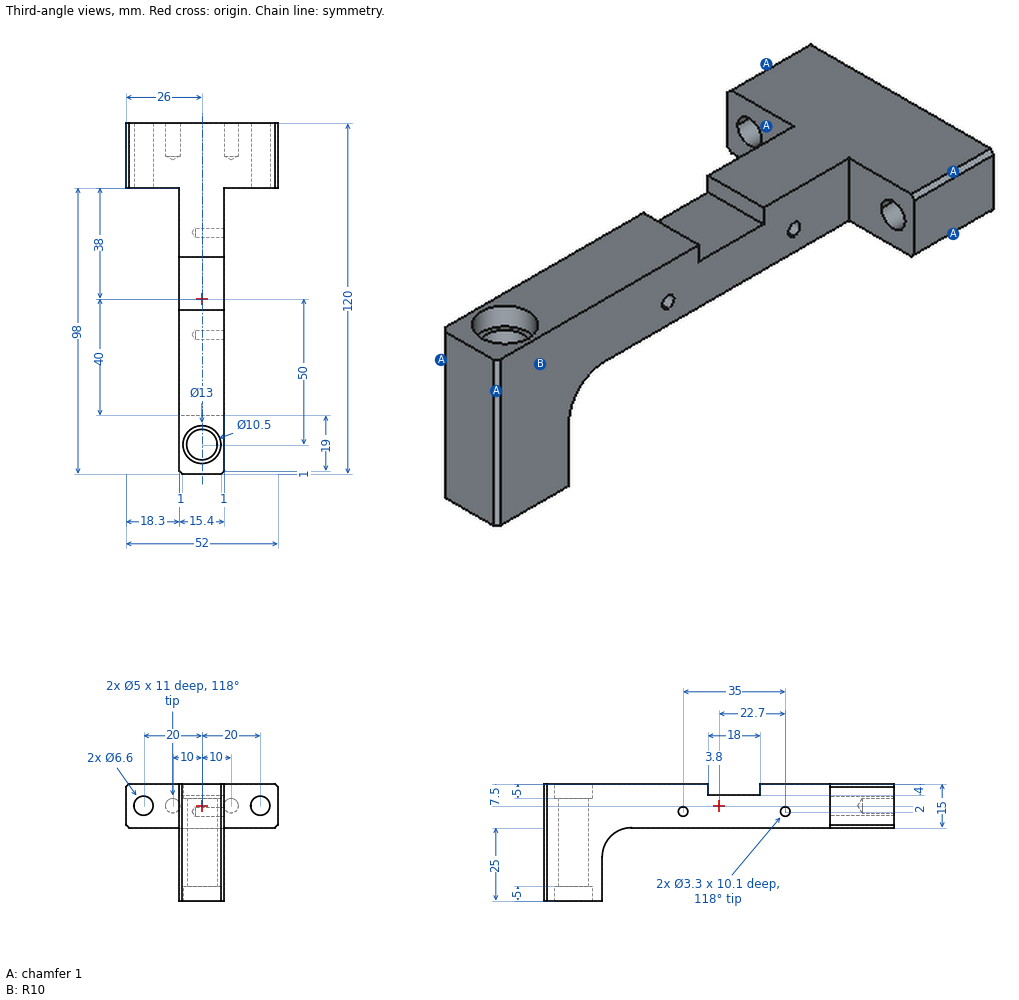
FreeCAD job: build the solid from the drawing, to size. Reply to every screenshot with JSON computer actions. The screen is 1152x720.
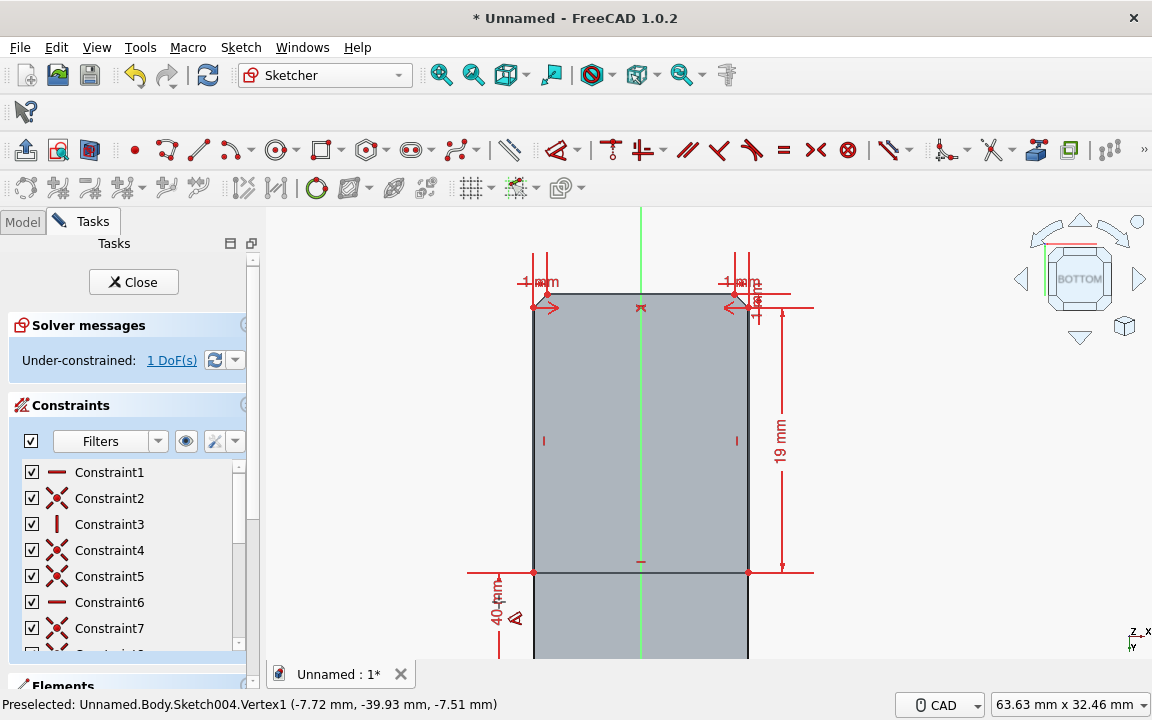
{"action": "left_click", "coordinate": [598, 573]}
{"action": "left_click", "coordinate": [592, 607]}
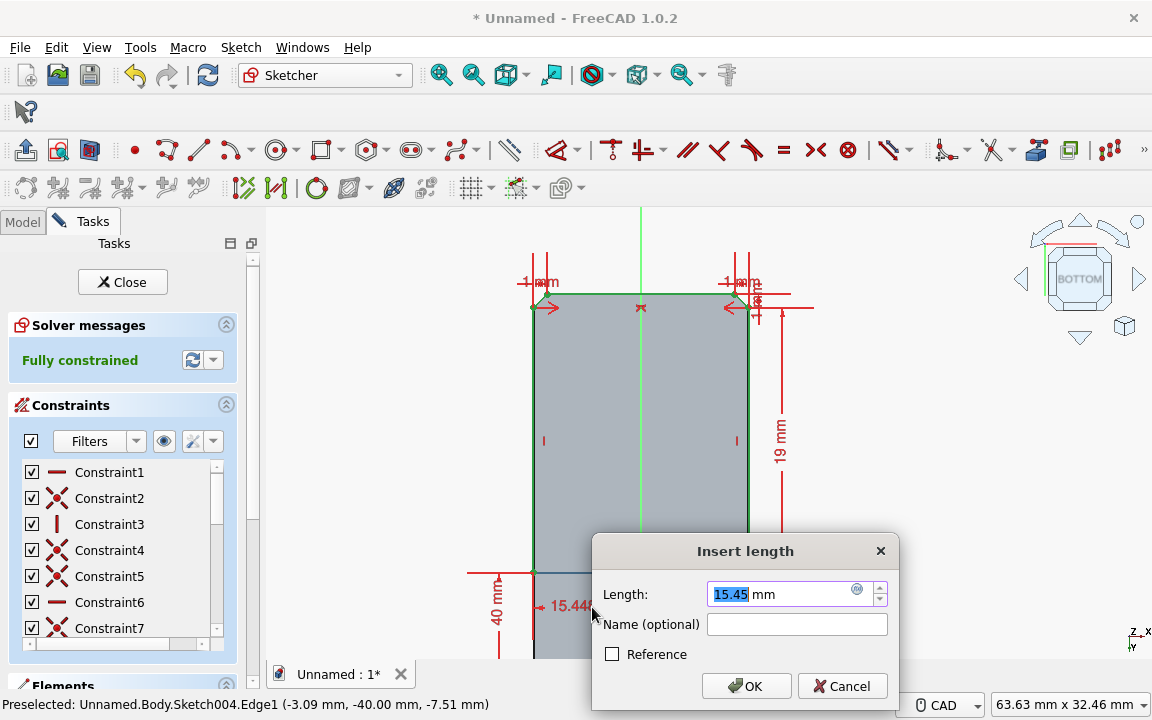
{"action": "type", "text": "15.4"}
{"action": "key", "text": "Return"}
{"action": "key", "text": "Escape"}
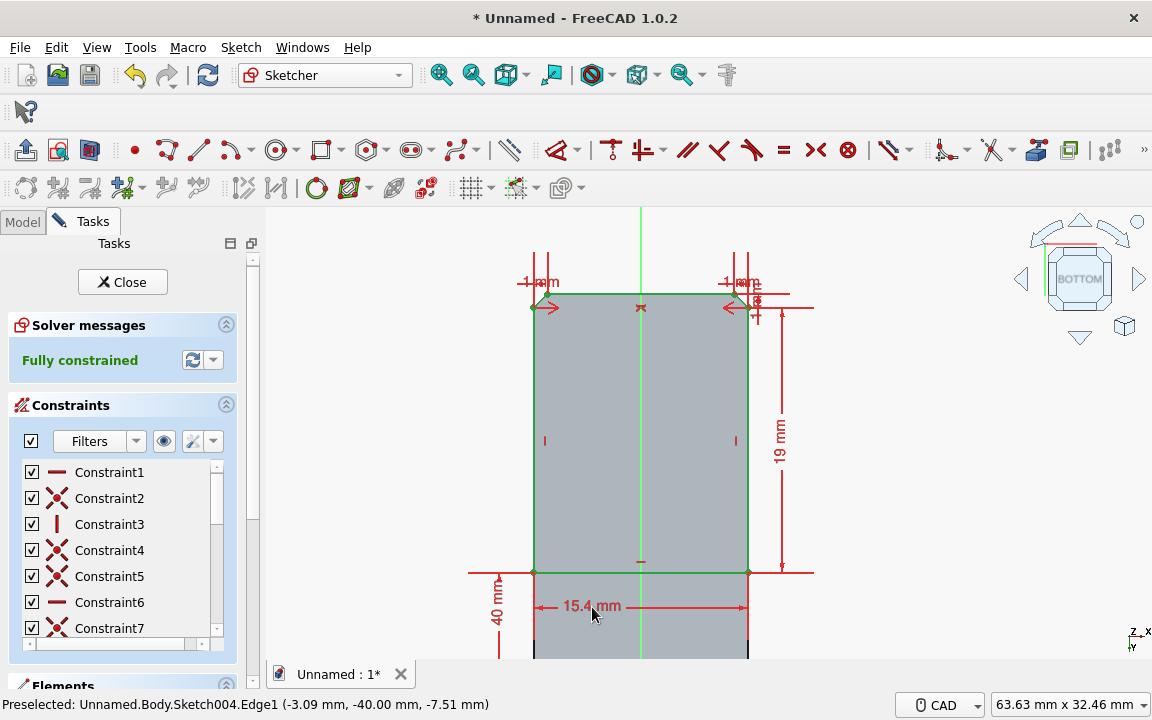
{"action": "left_click", "coordinate": [123, 282]}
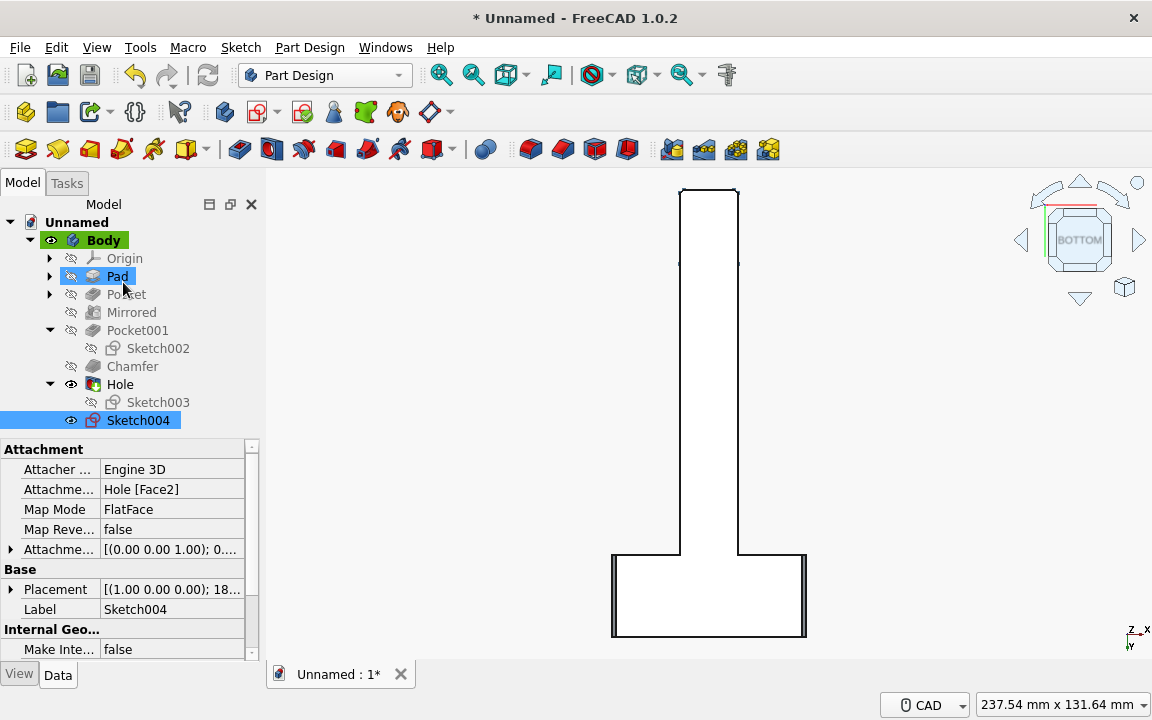
{"action": "left_click", "coordinate": [26, 150]}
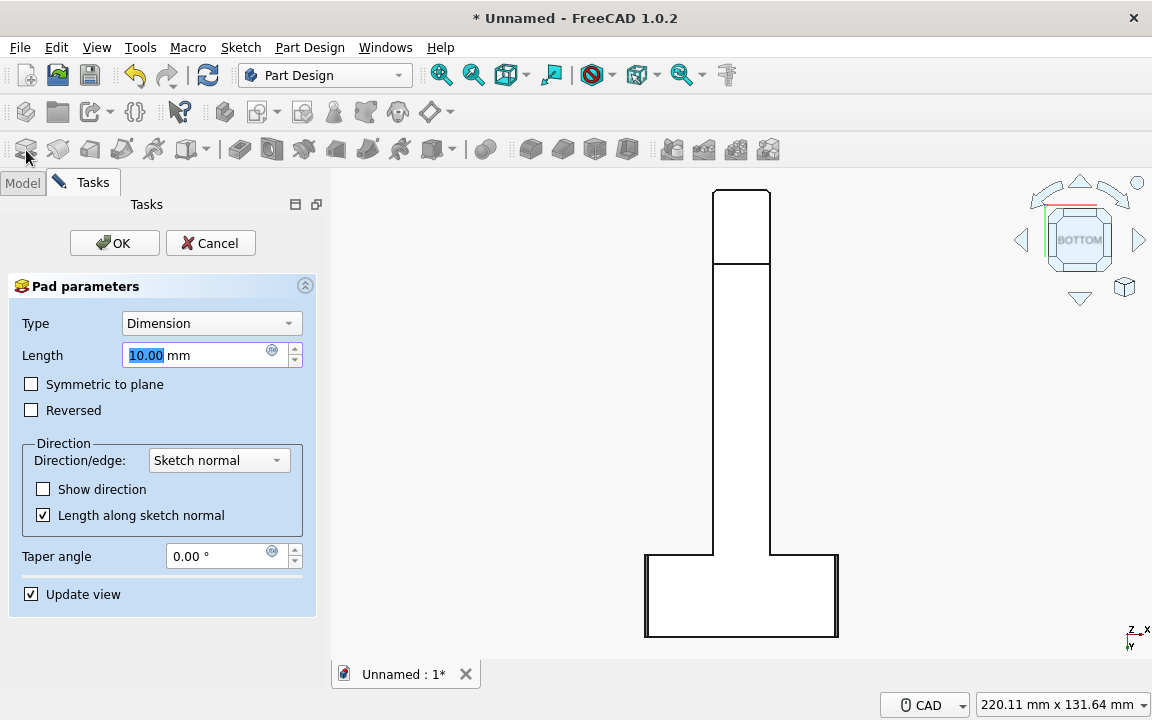
{"action": "type", "text": "25"}
{"action": "key", "text": "Tab"}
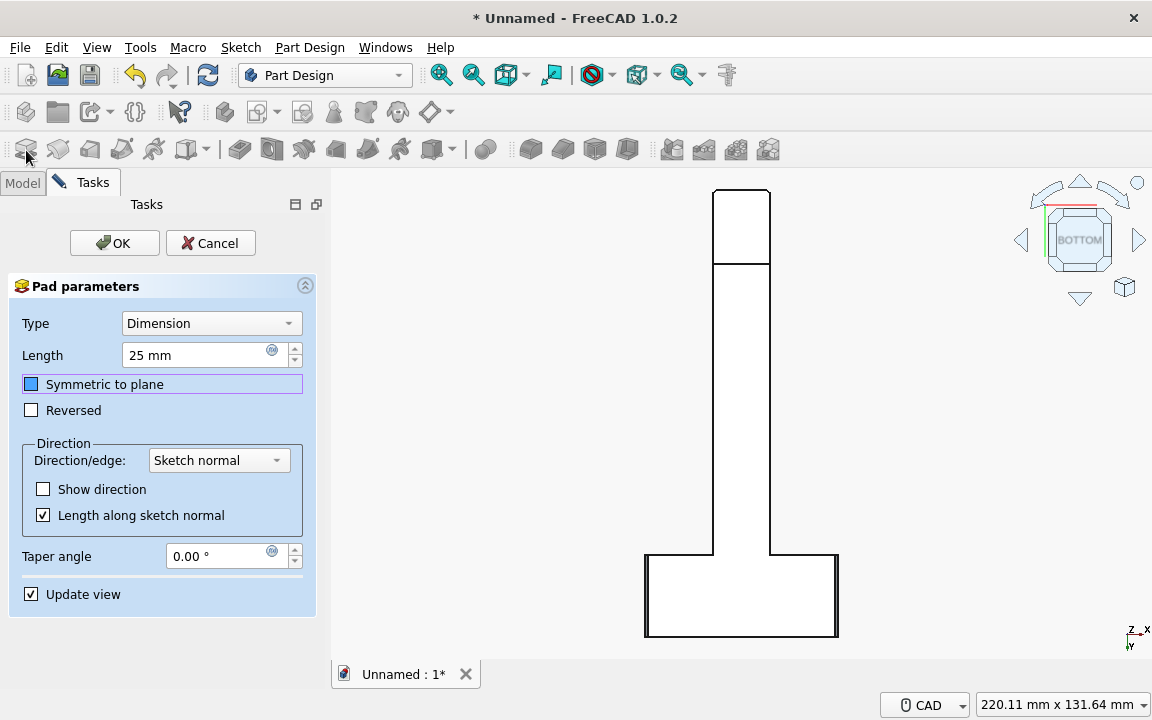
{"action": "left_click", "coordinate": [115, 243]}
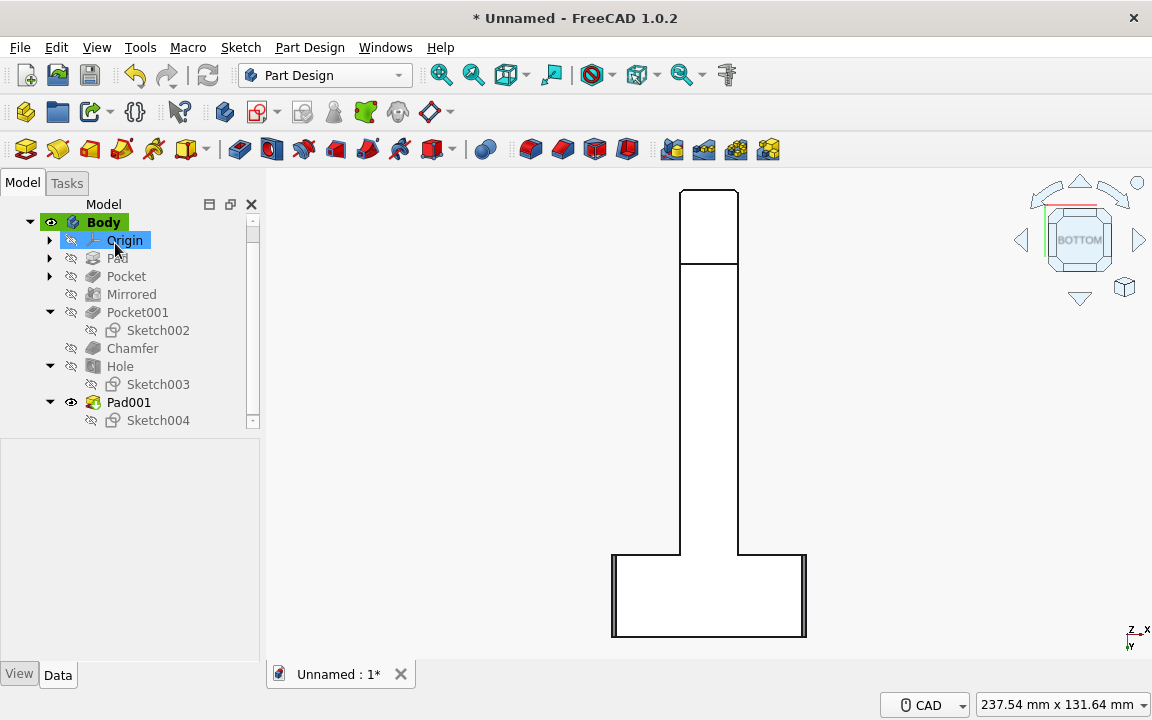
{"action": "key", "text": "0"}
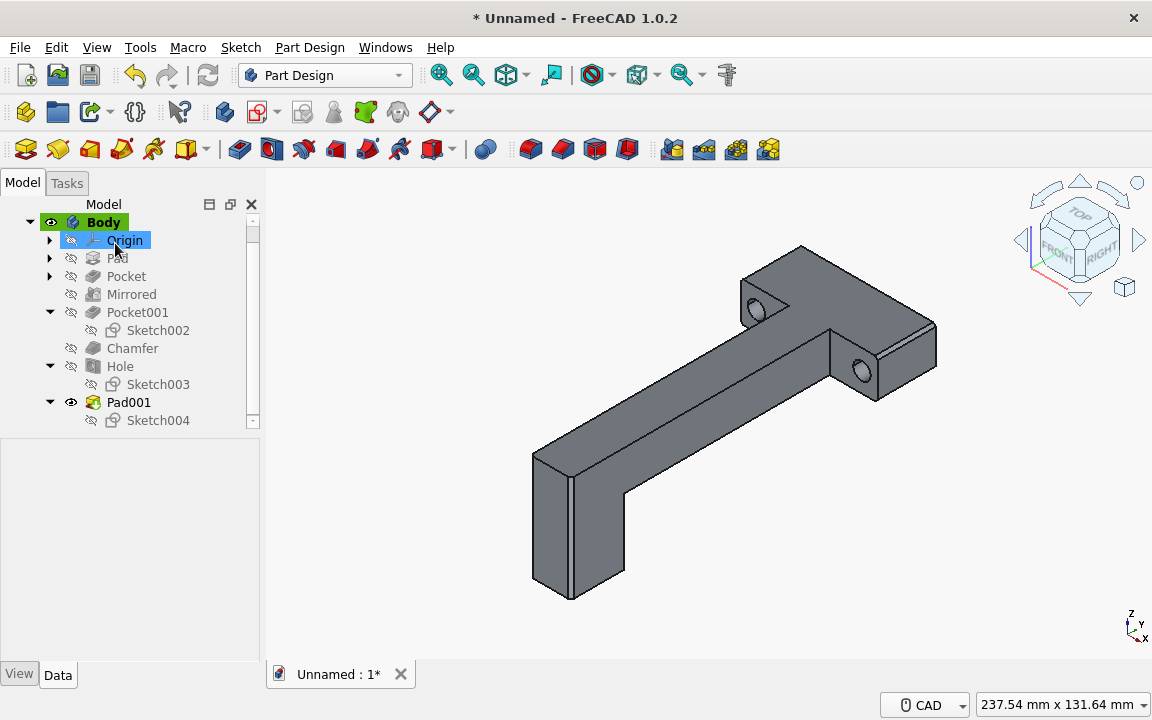
{"action": "key", "text": "2"}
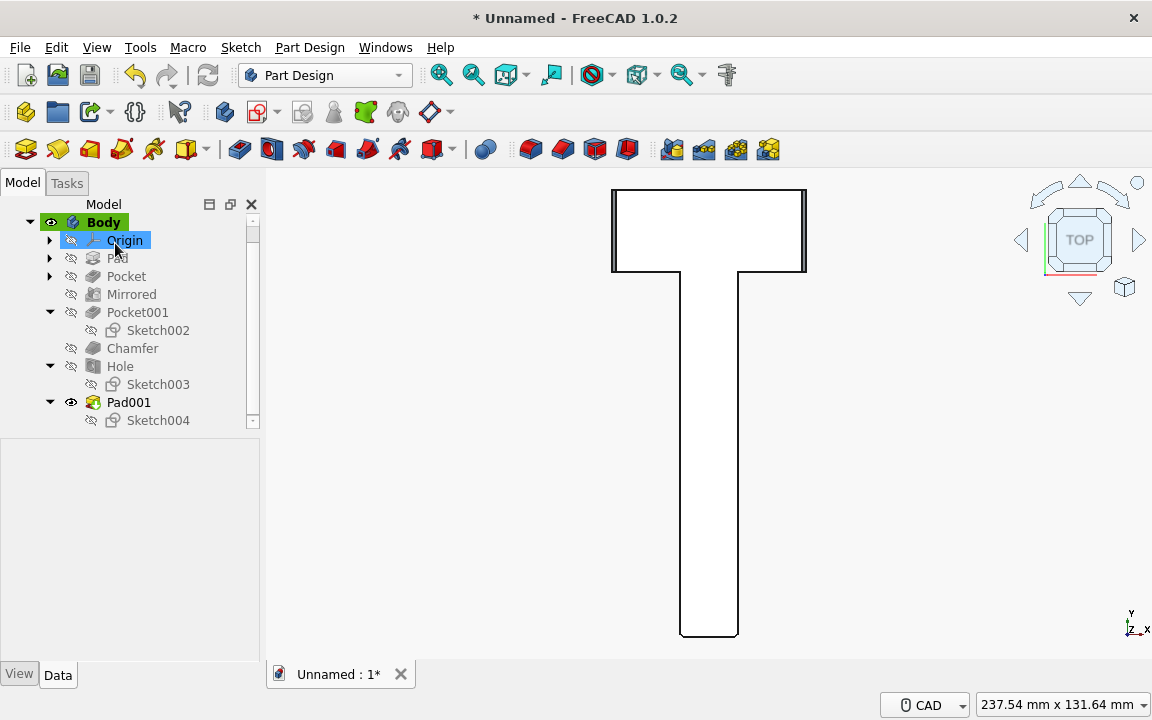
{"action": "key", "text": "1"}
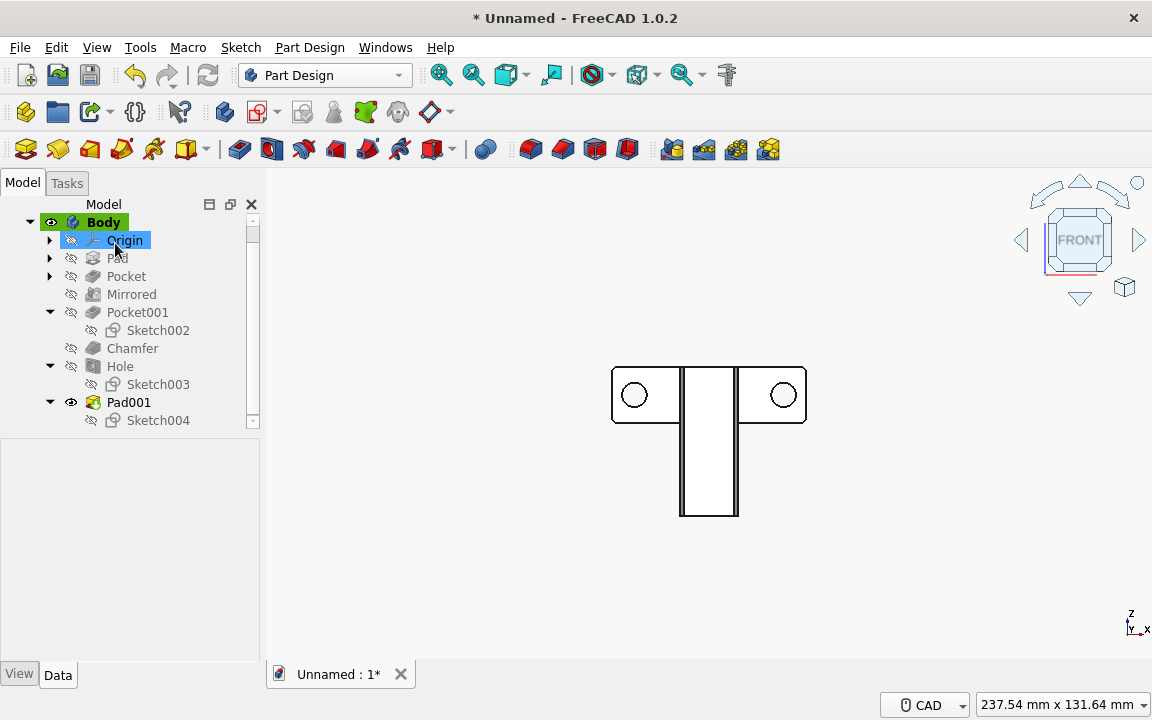
{"action": "left_click", "coordinate": [442, 76]}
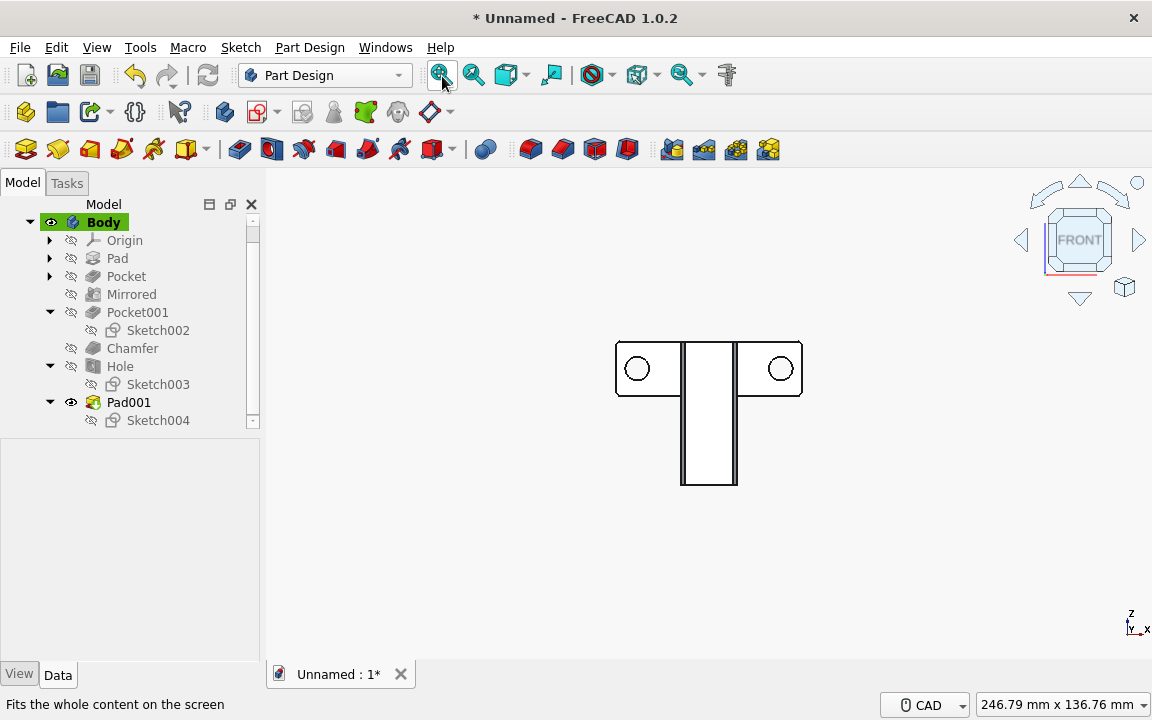
{"action": "key", "text": "3"}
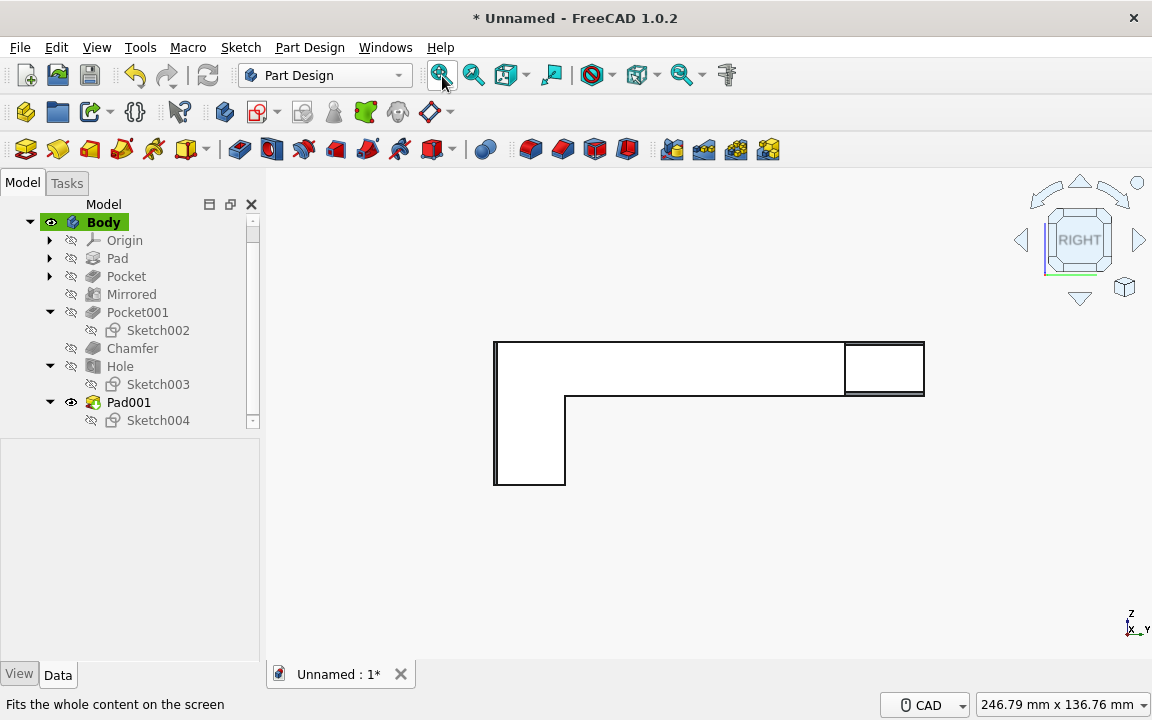
{"action": "key", "text": "5"}